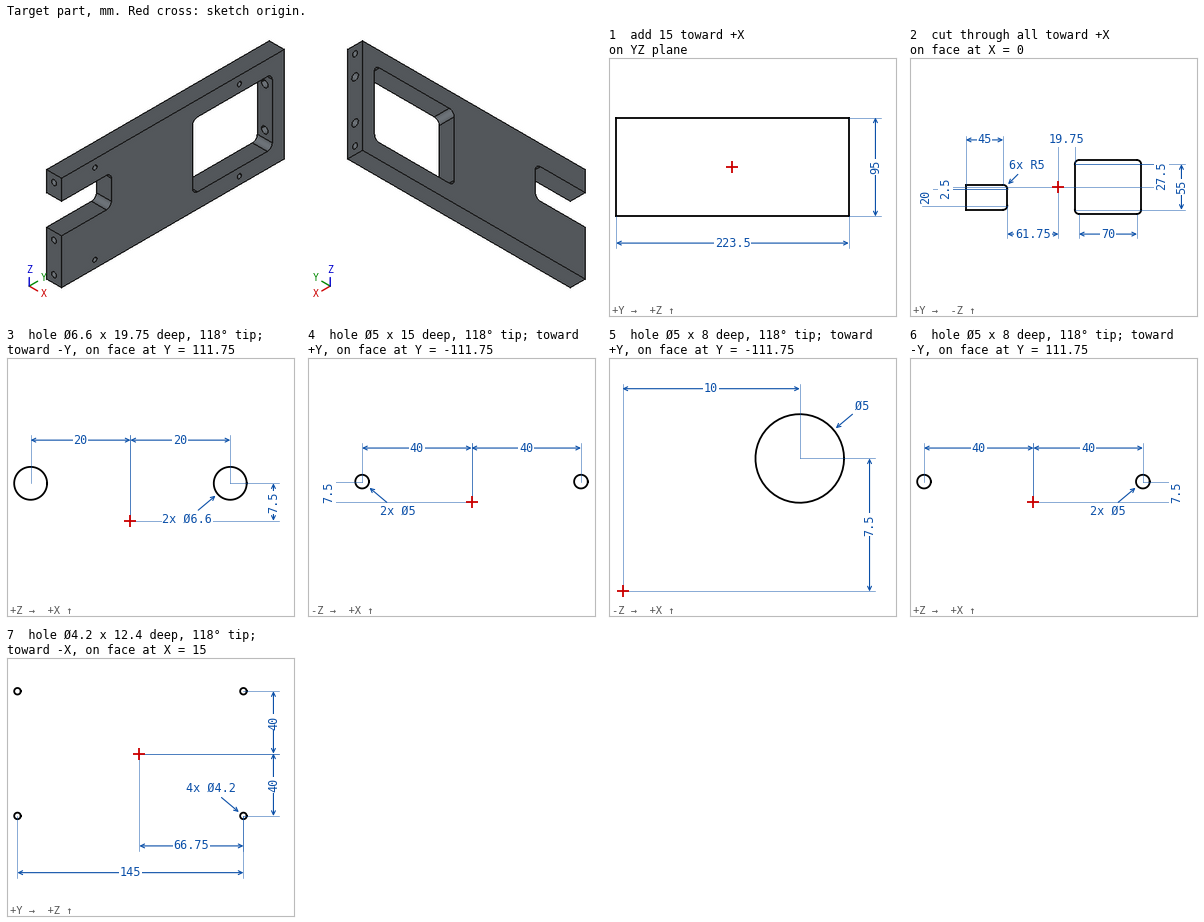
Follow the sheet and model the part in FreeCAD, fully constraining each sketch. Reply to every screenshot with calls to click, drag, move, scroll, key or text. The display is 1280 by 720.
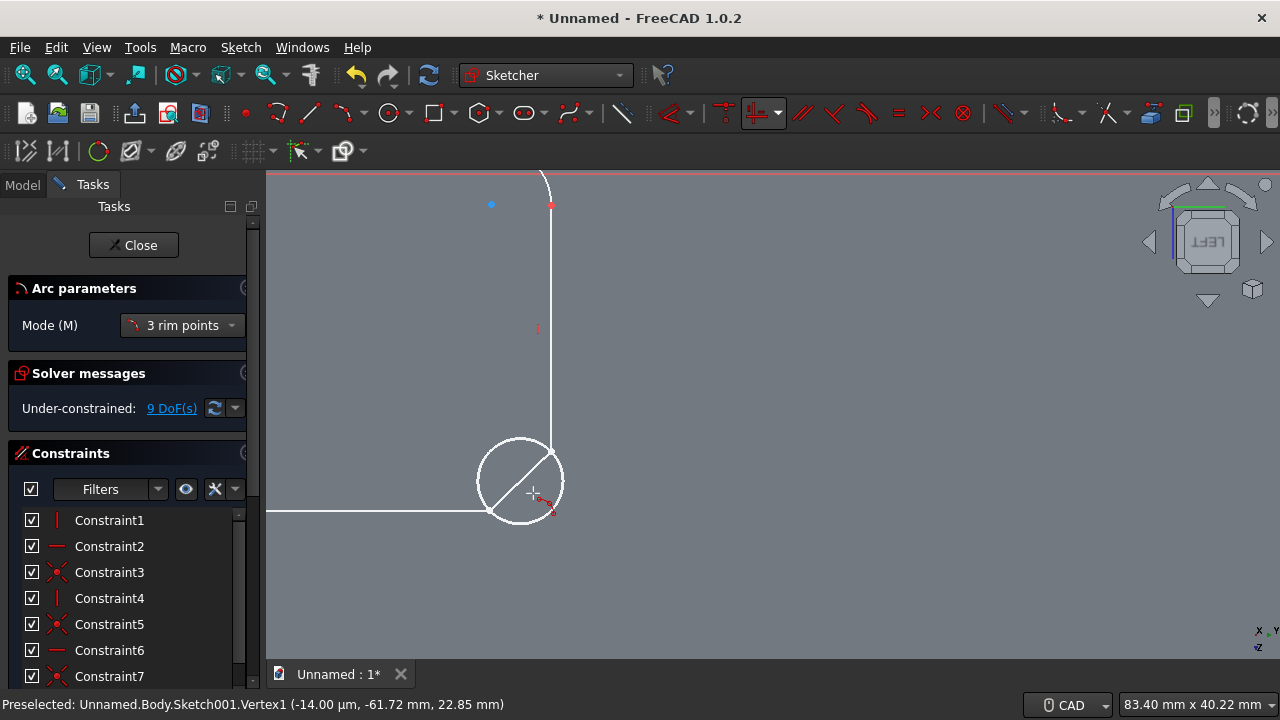
click(533, 490)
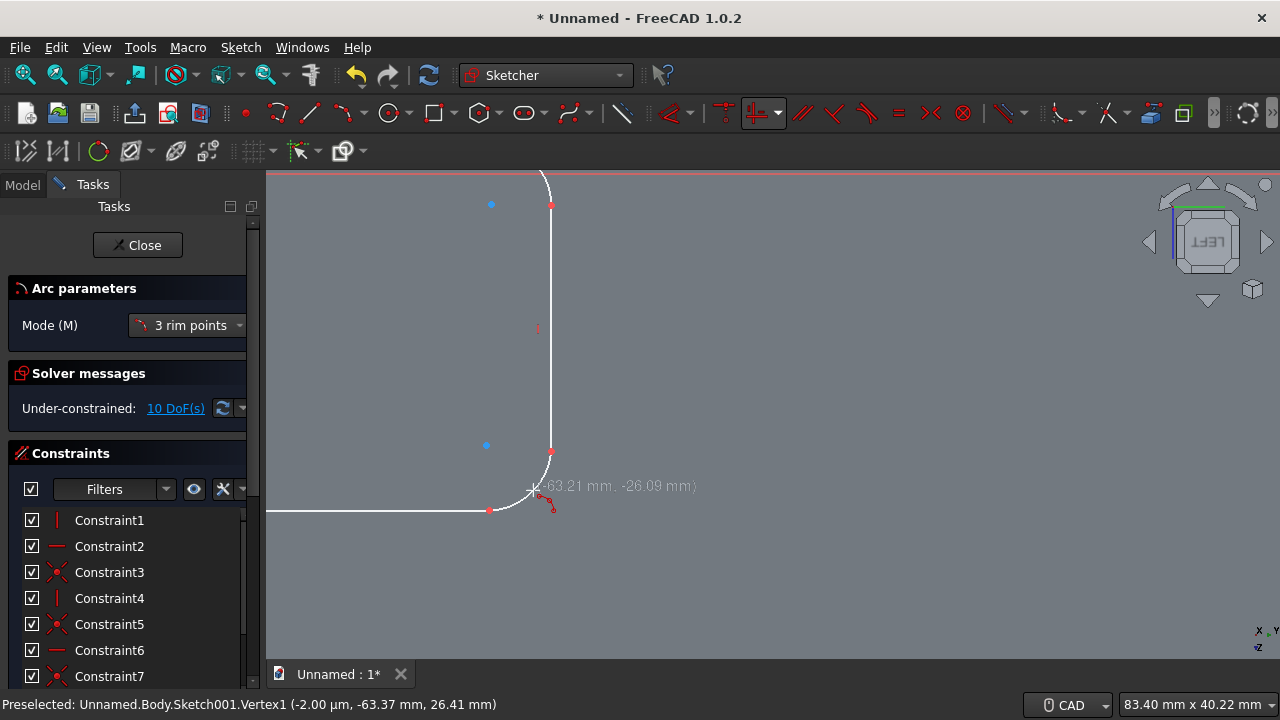
click(310, 114)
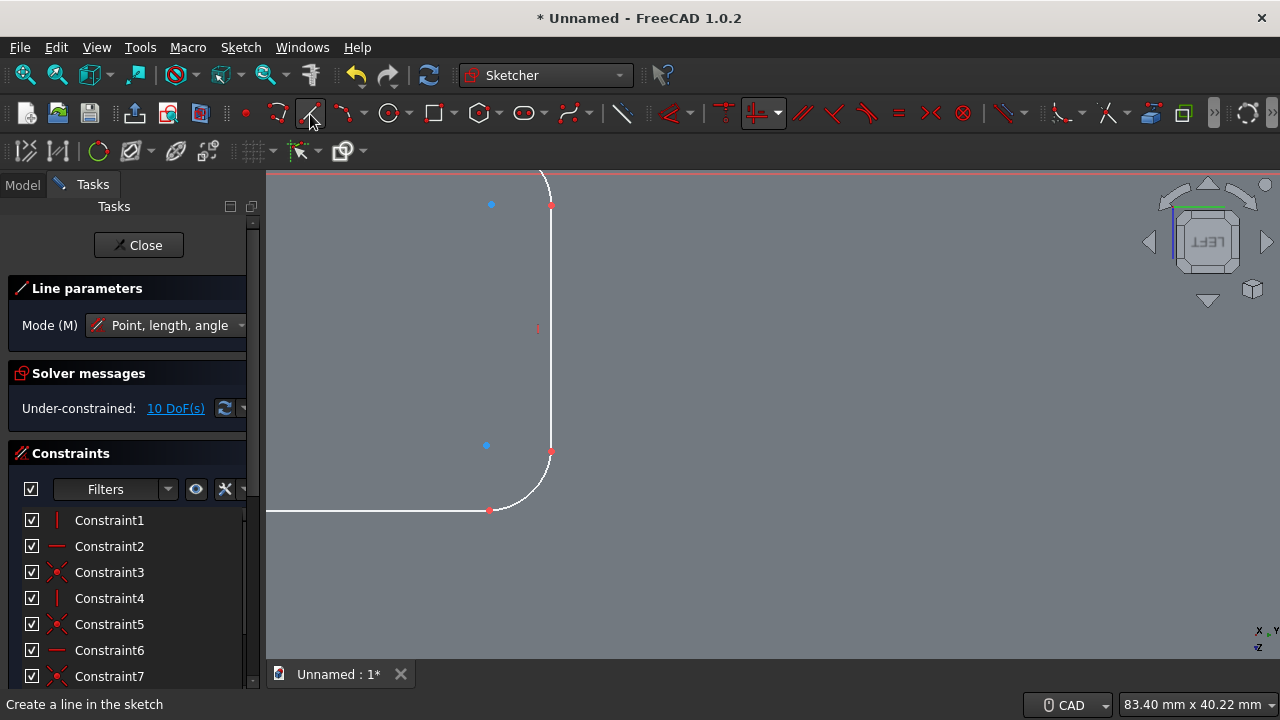
scroll(533, 493, down, 7)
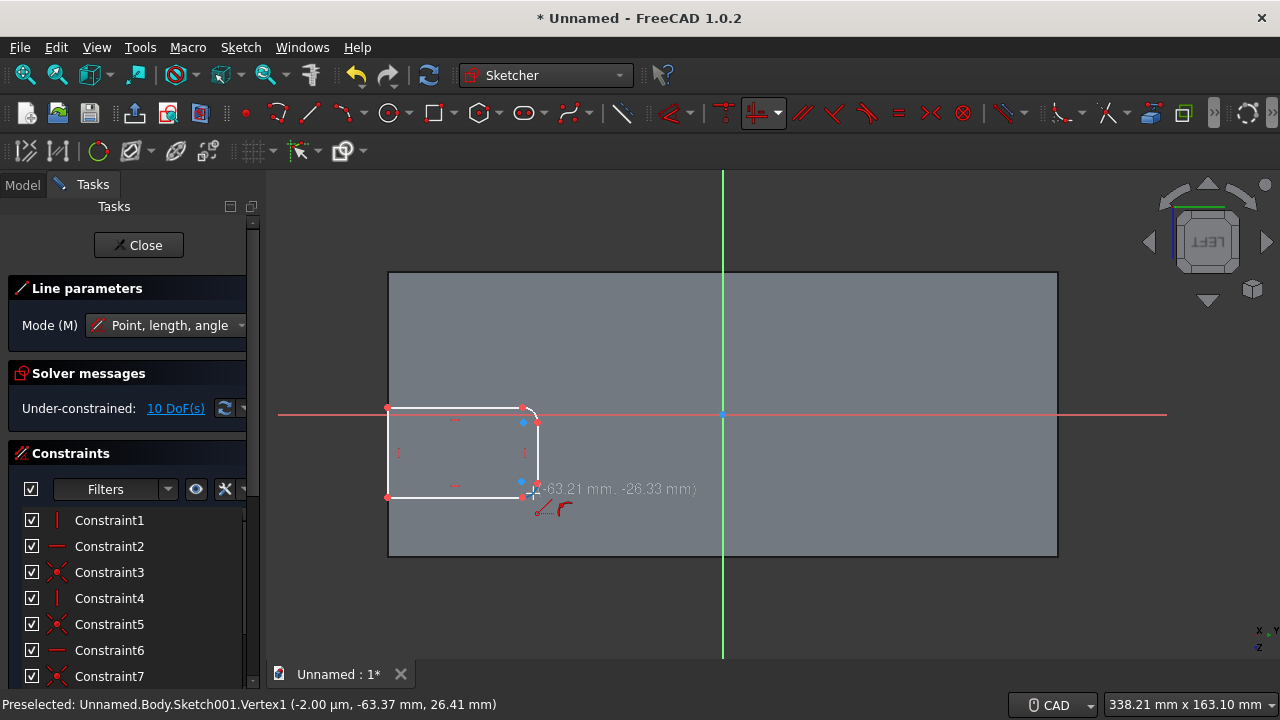
click(782, 332)
click(782, 497)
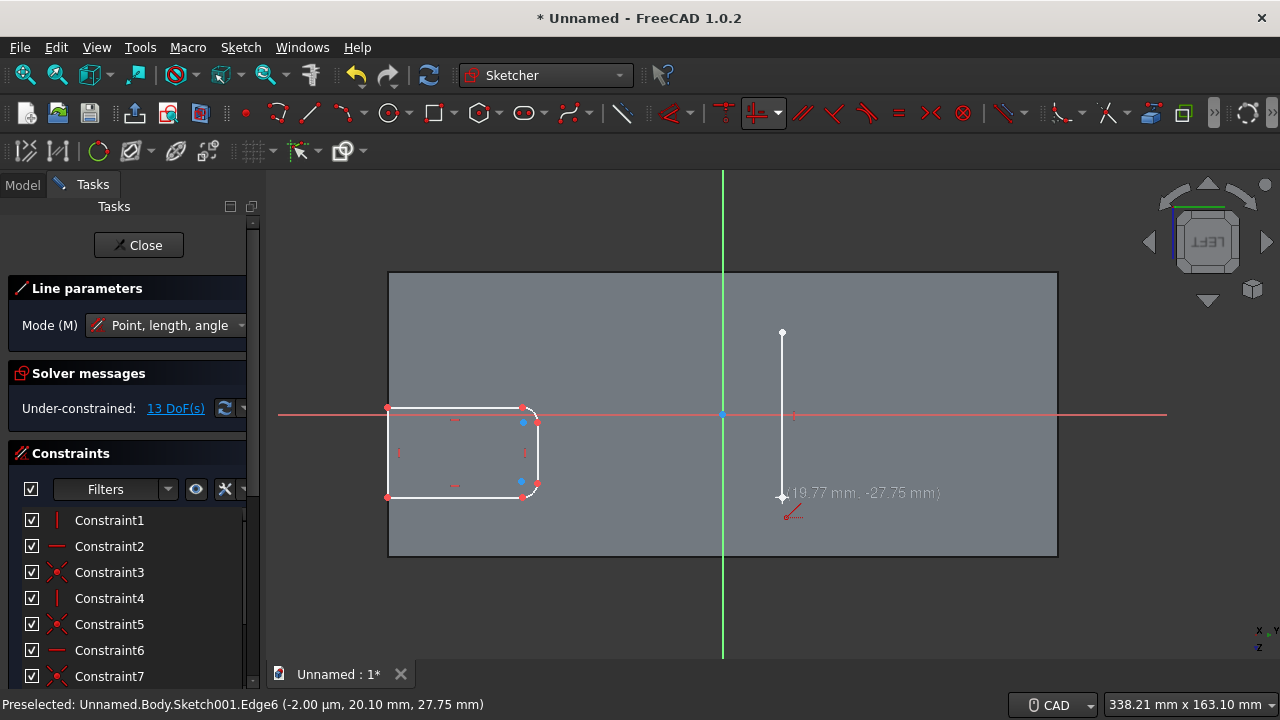
click(797, 512)
click(1007, 512)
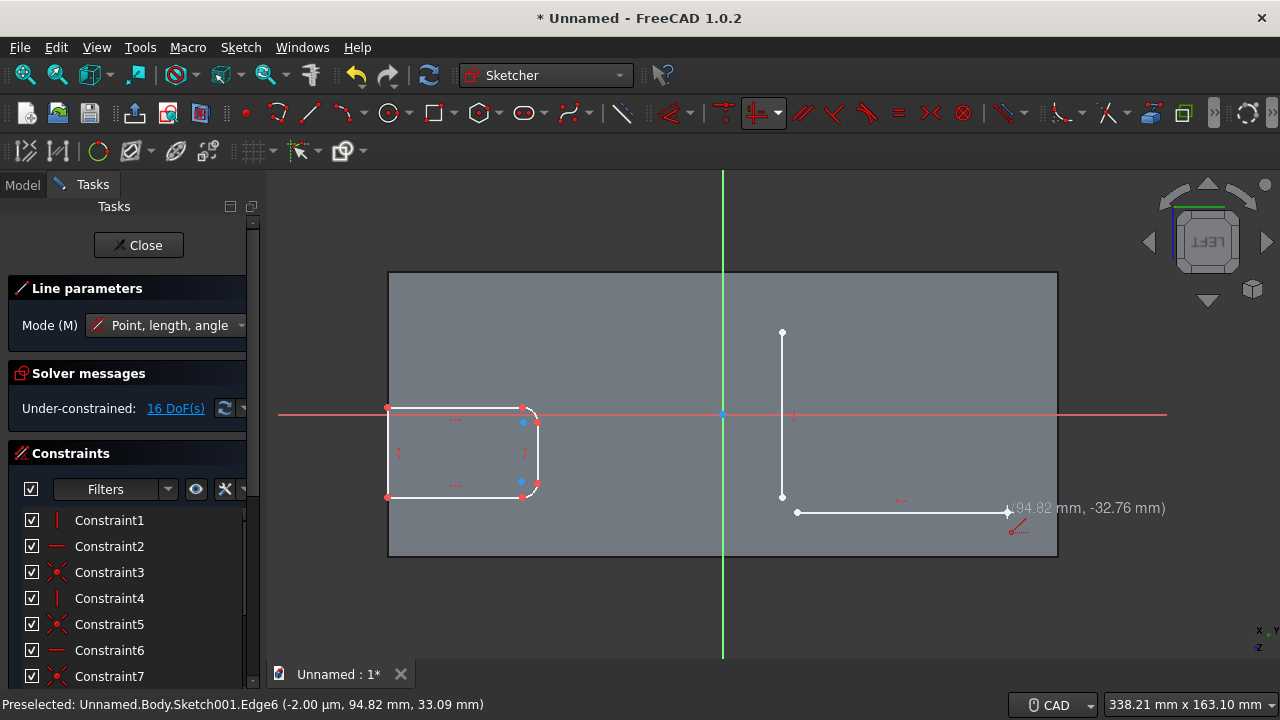
click(1022, 497)
click(1022, 332)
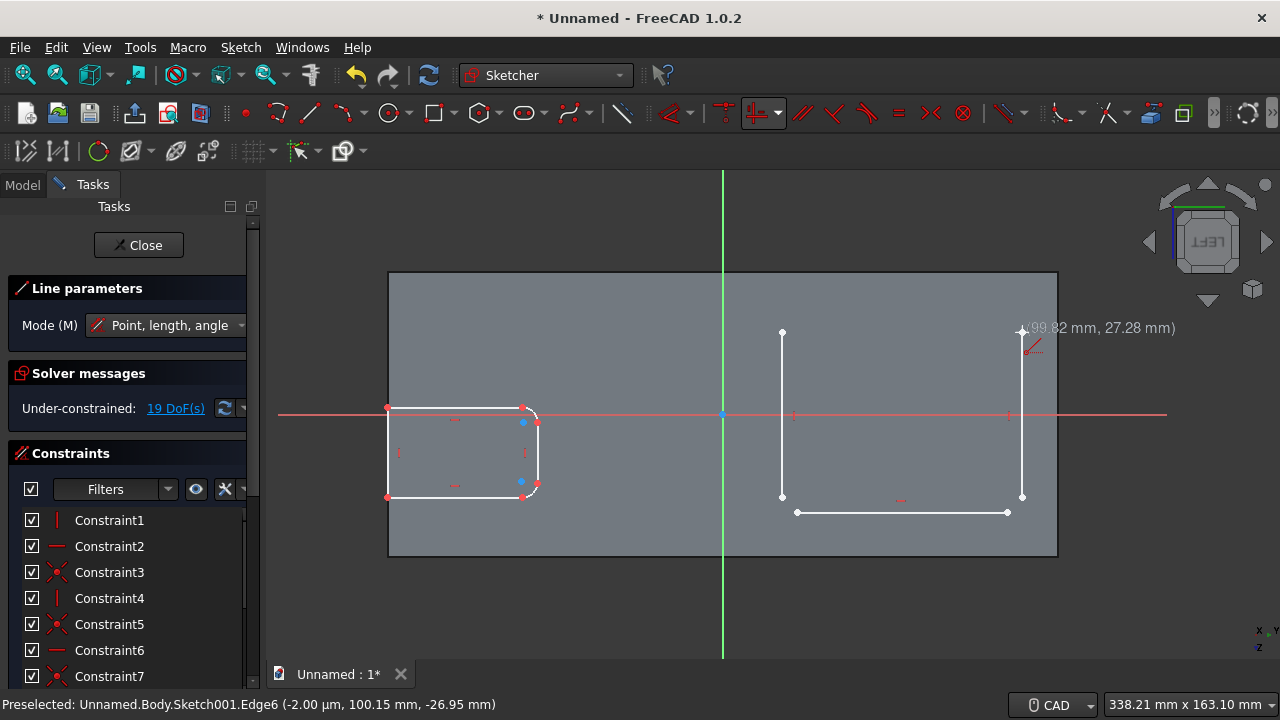
click(1007, 317)
click(797, 317)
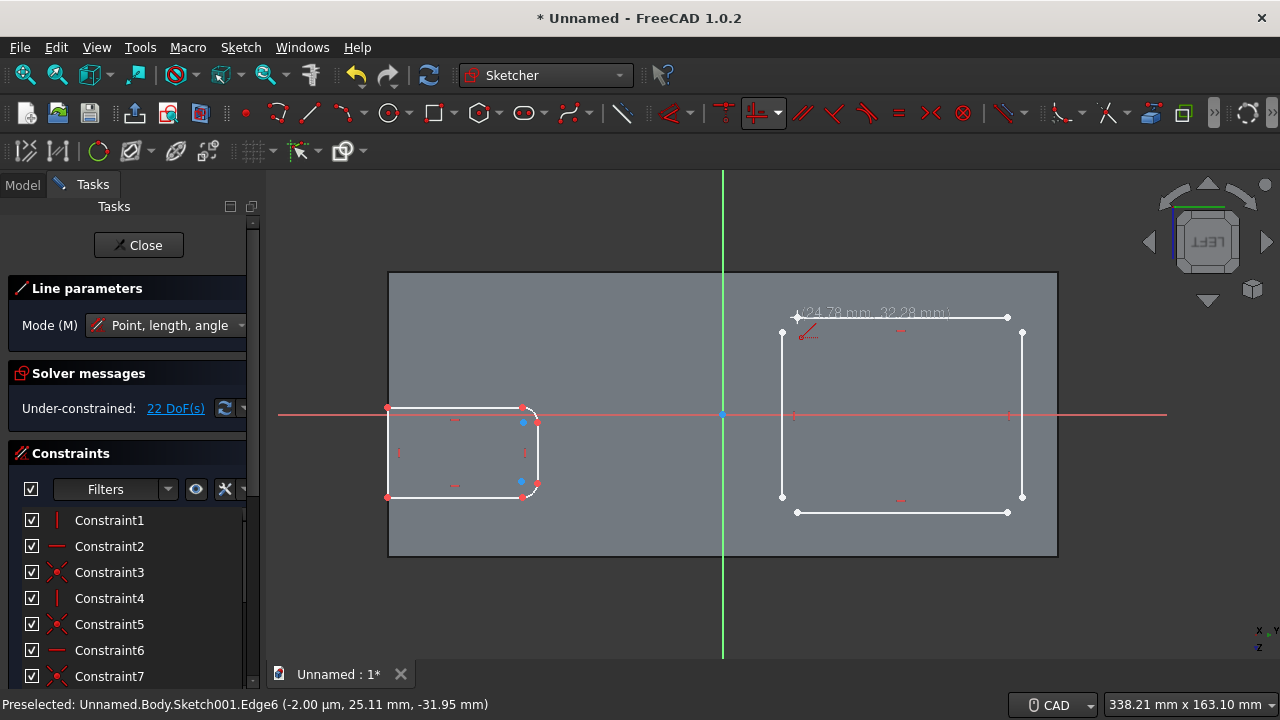
click(344, 114)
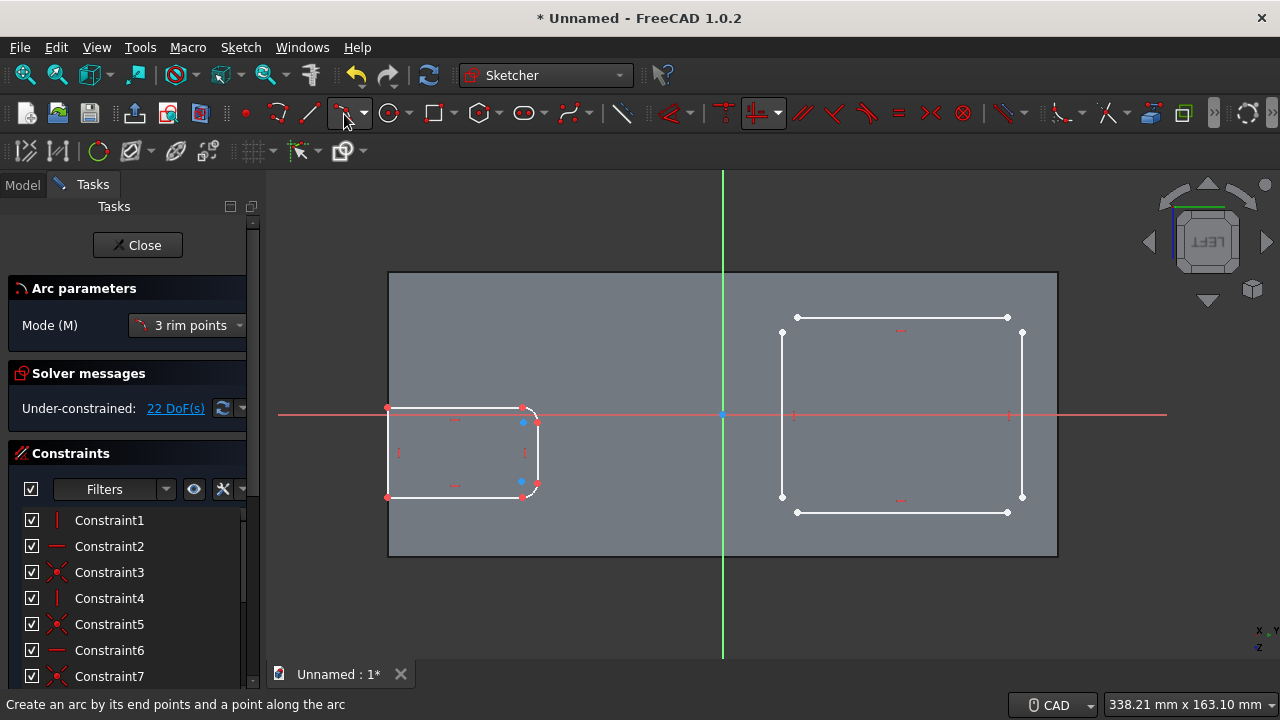
click(782, 498)
click(797, 513)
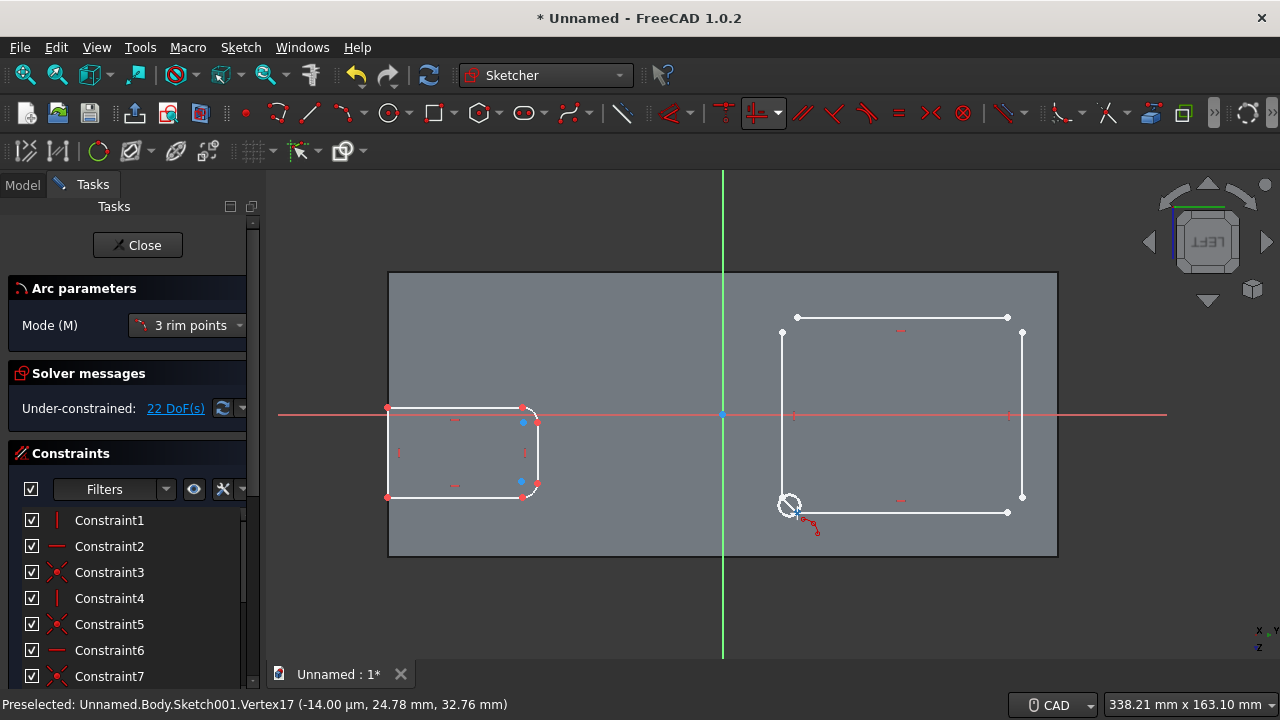
scroll(786, 508, up, 7)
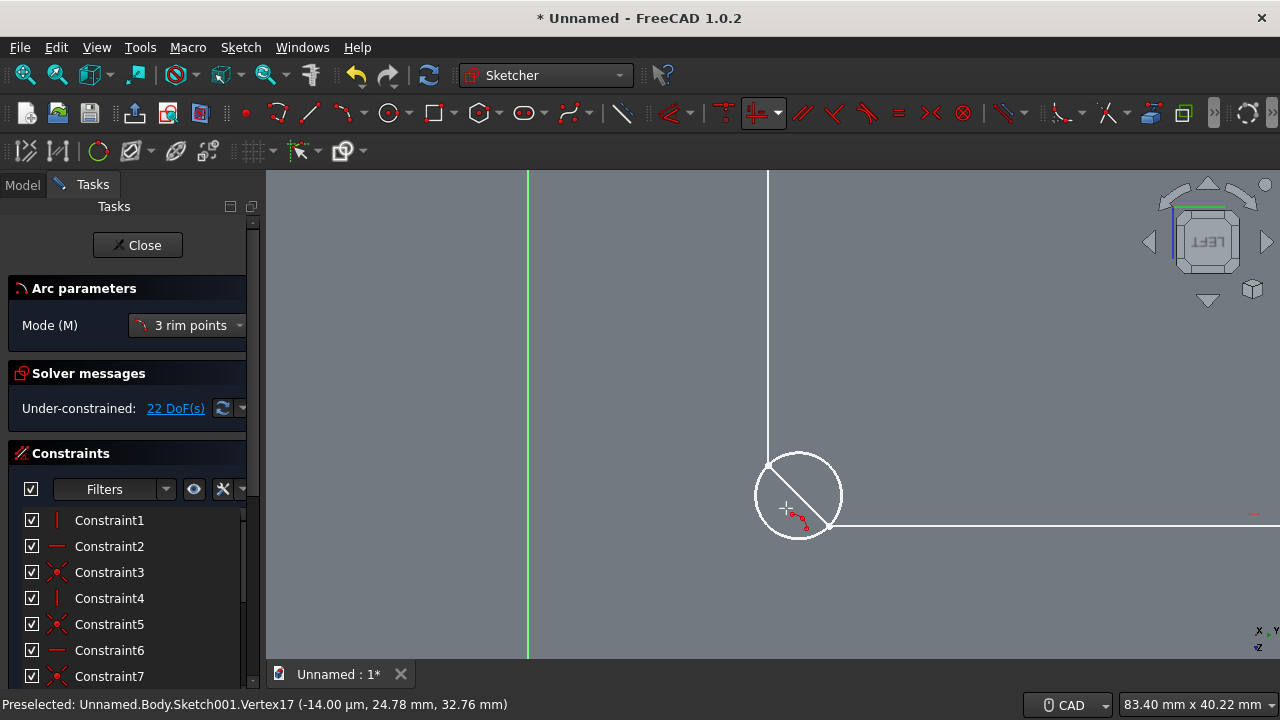
click(786, 505)